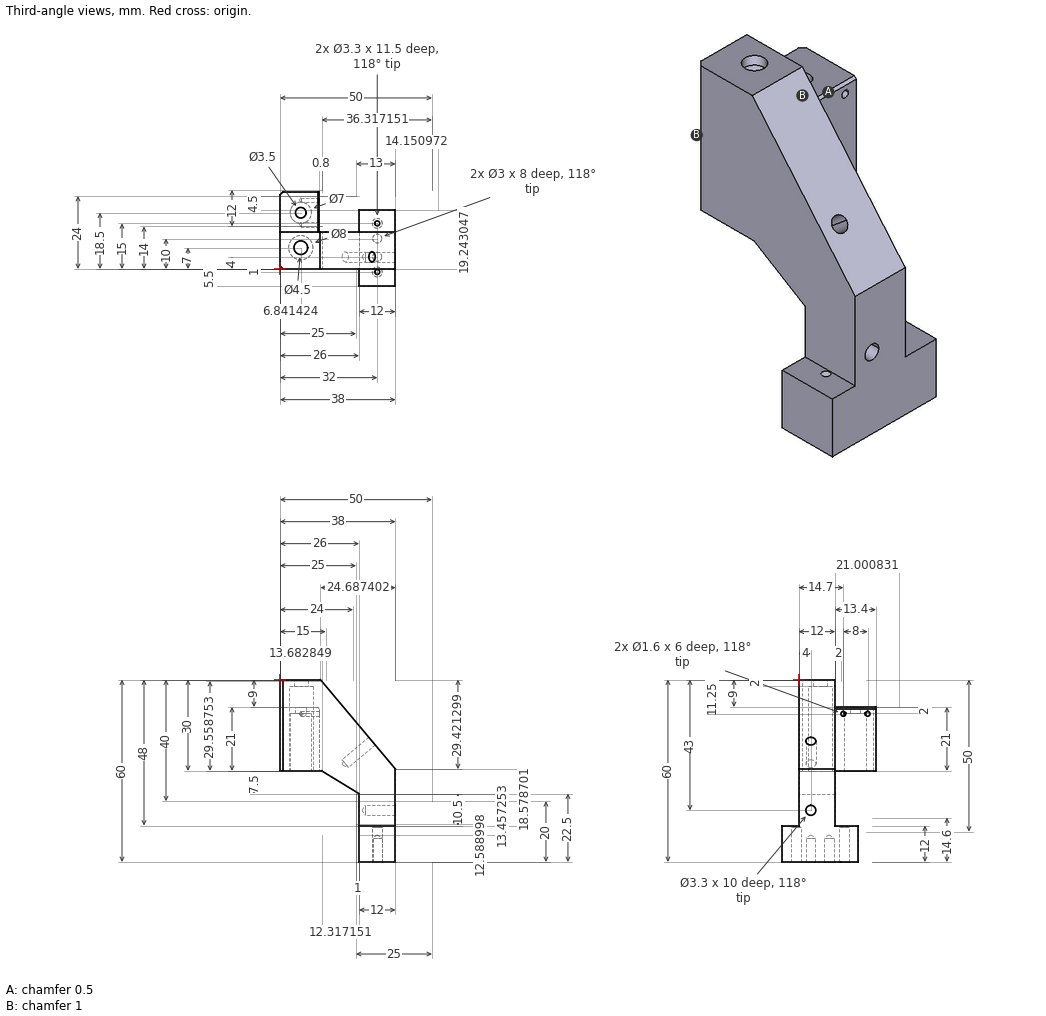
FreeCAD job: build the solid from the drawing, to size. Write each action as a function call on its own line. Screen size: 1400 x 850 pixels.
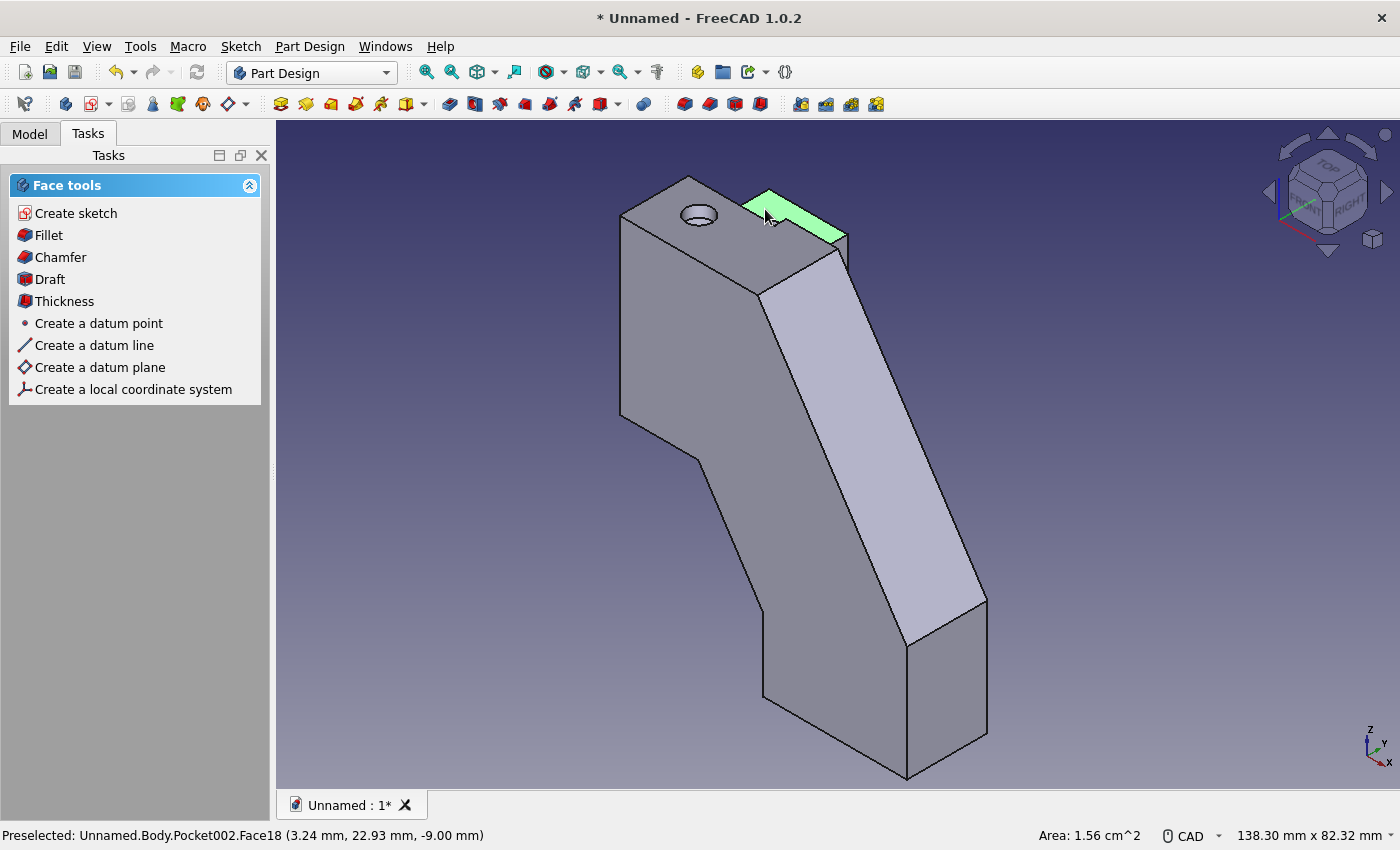
click(90, 104)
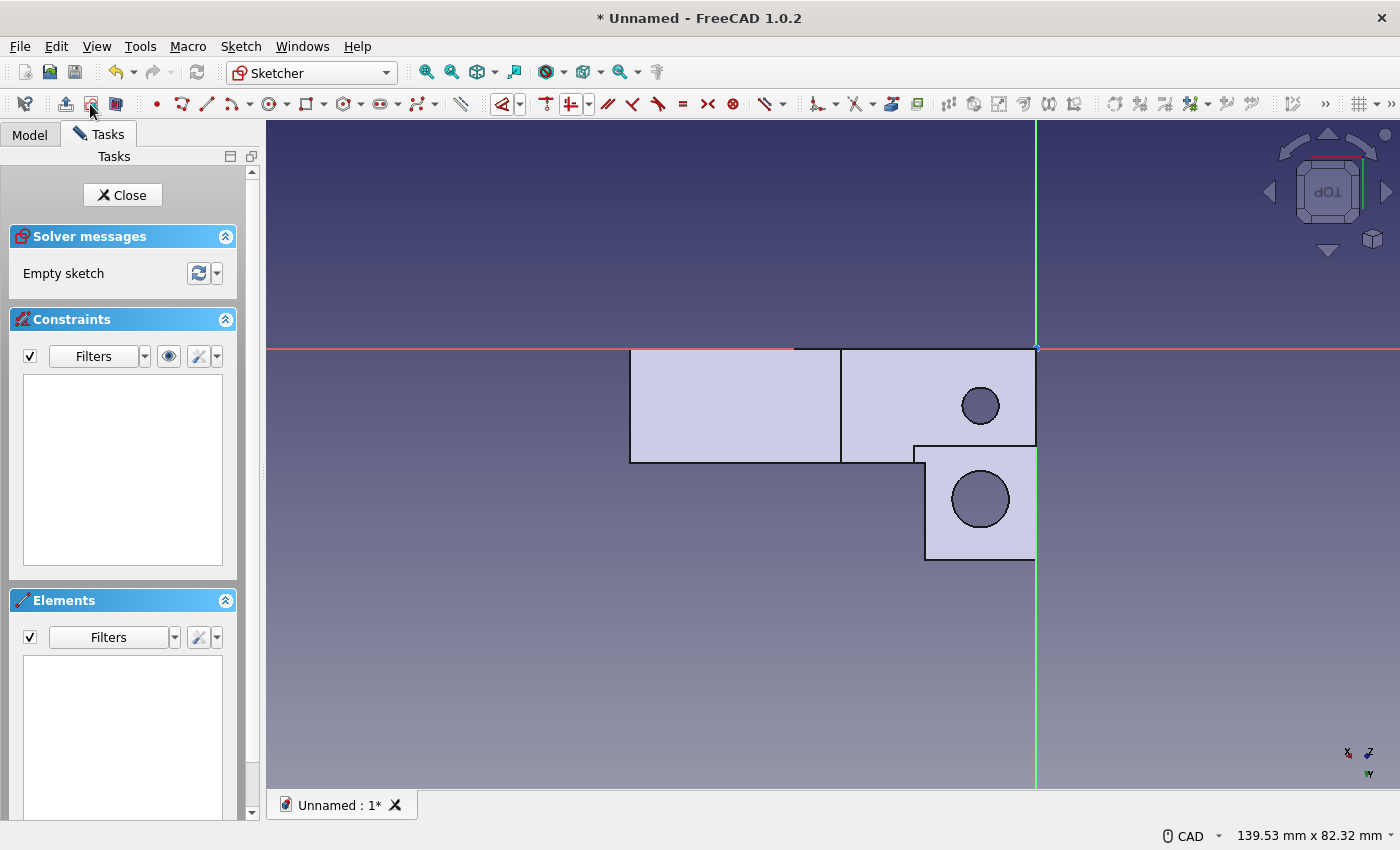
key(q)
key(s)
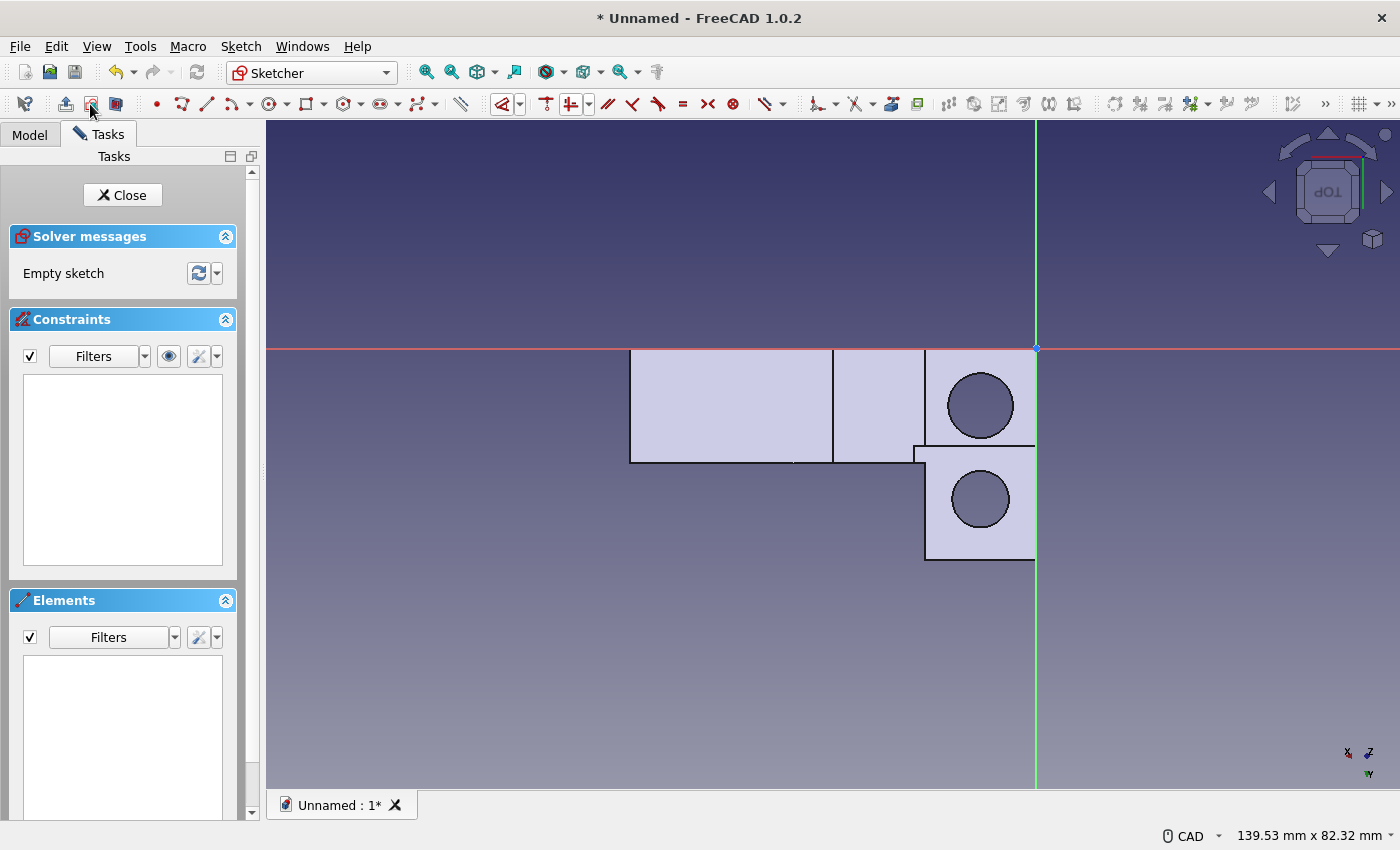
scroll(1014, 506, up, 10)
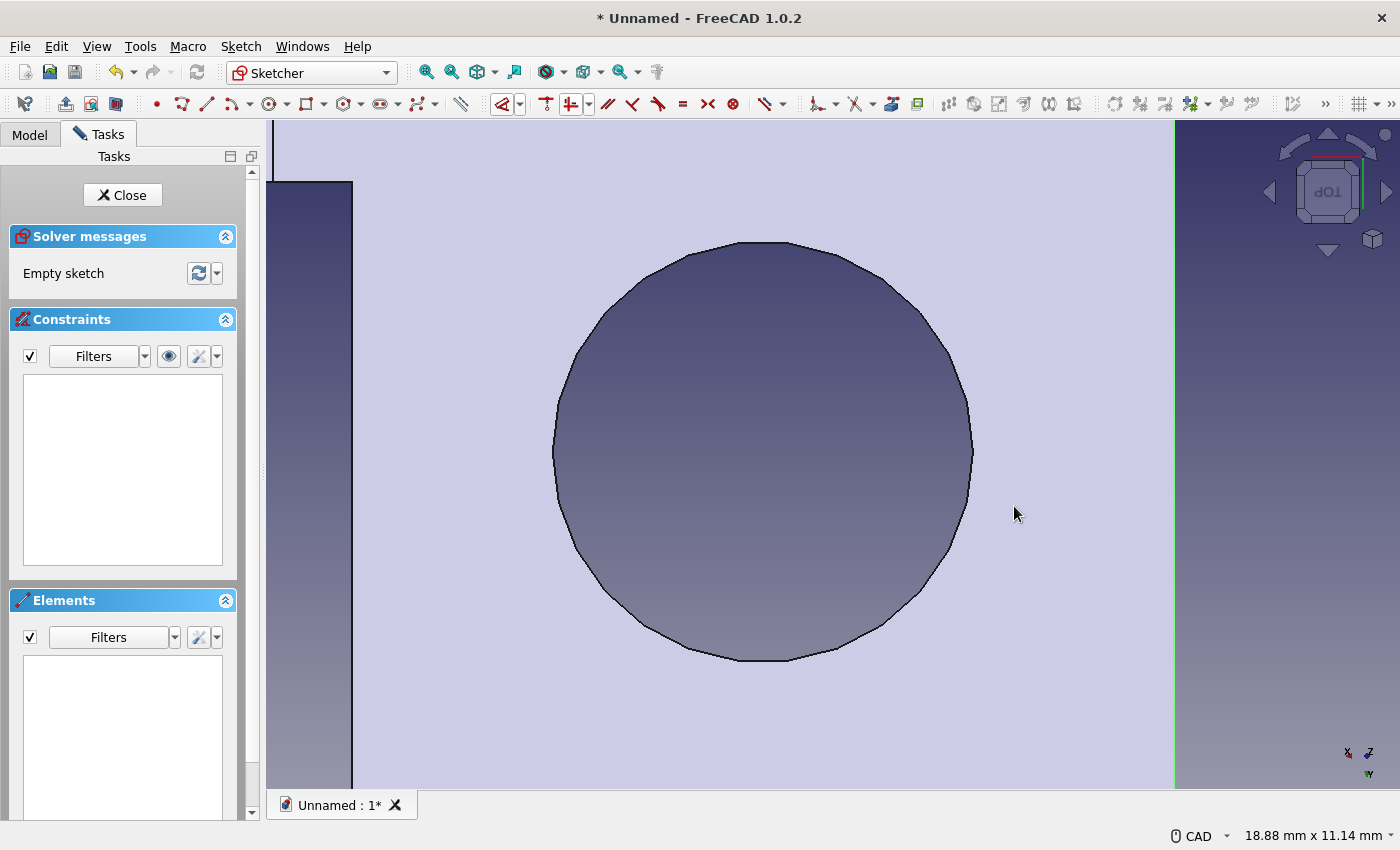
click(268, 104)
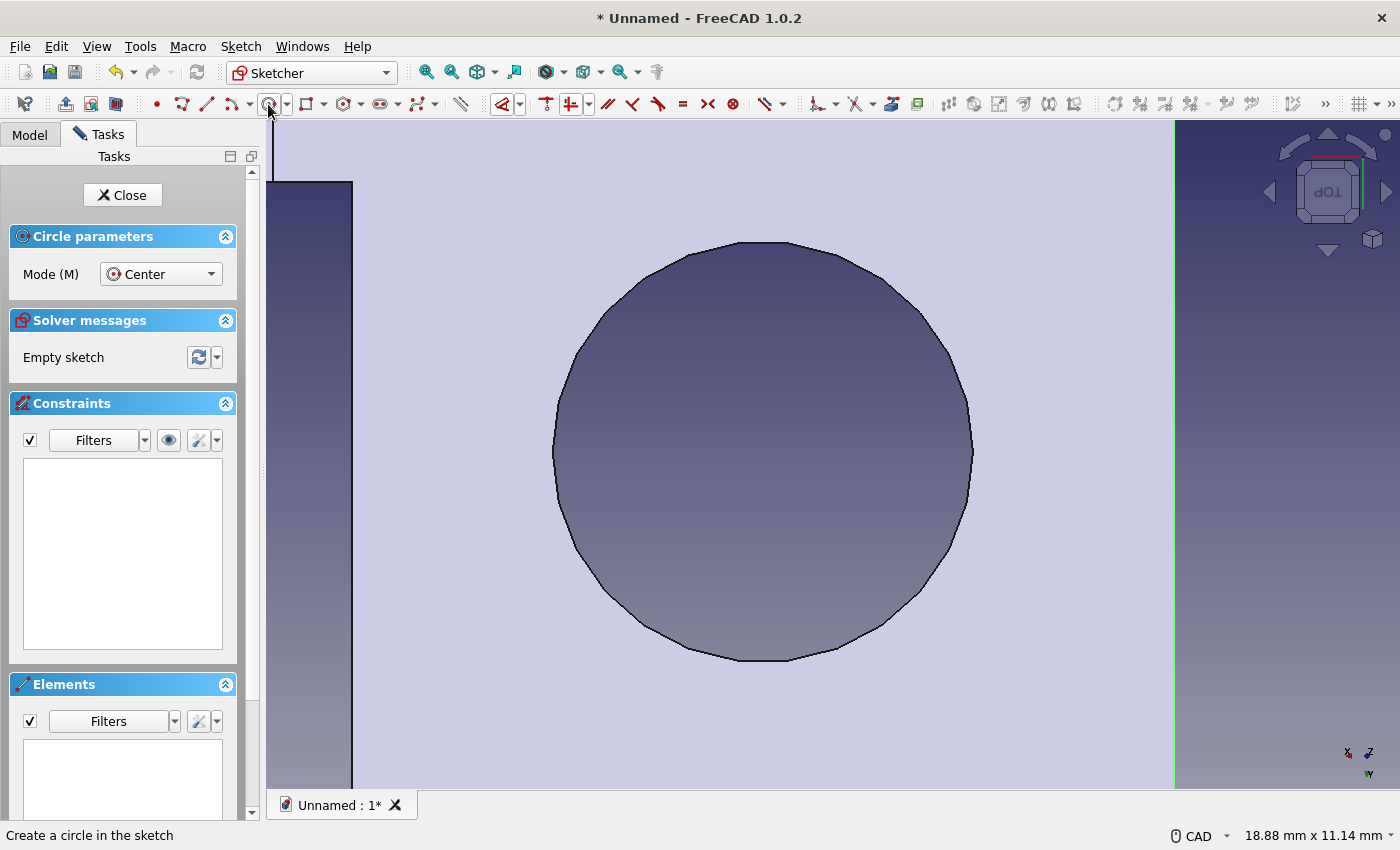
click(763, 452)
click(911, 303)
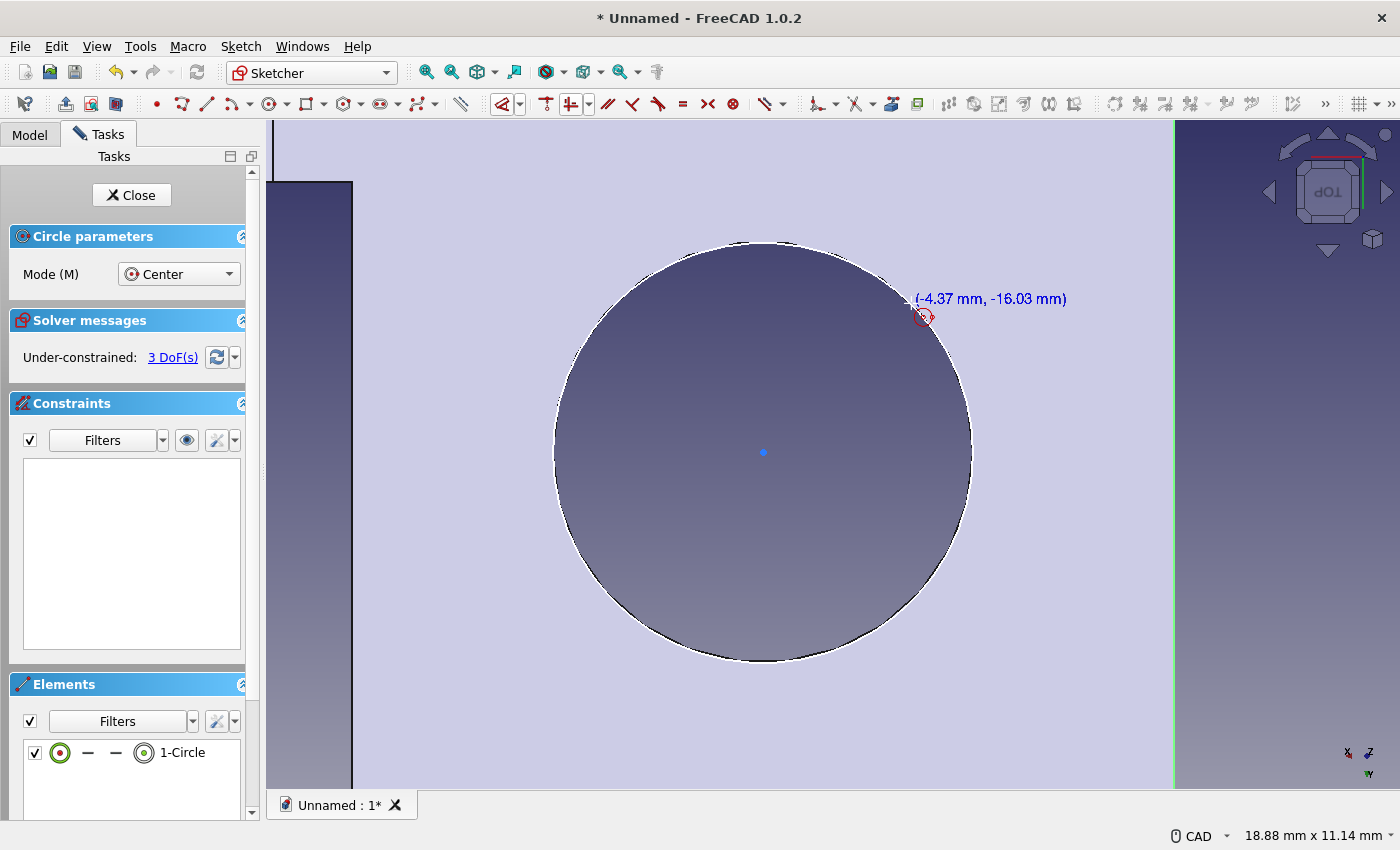
click(763, 453)
click(837, 378)
key(Escape)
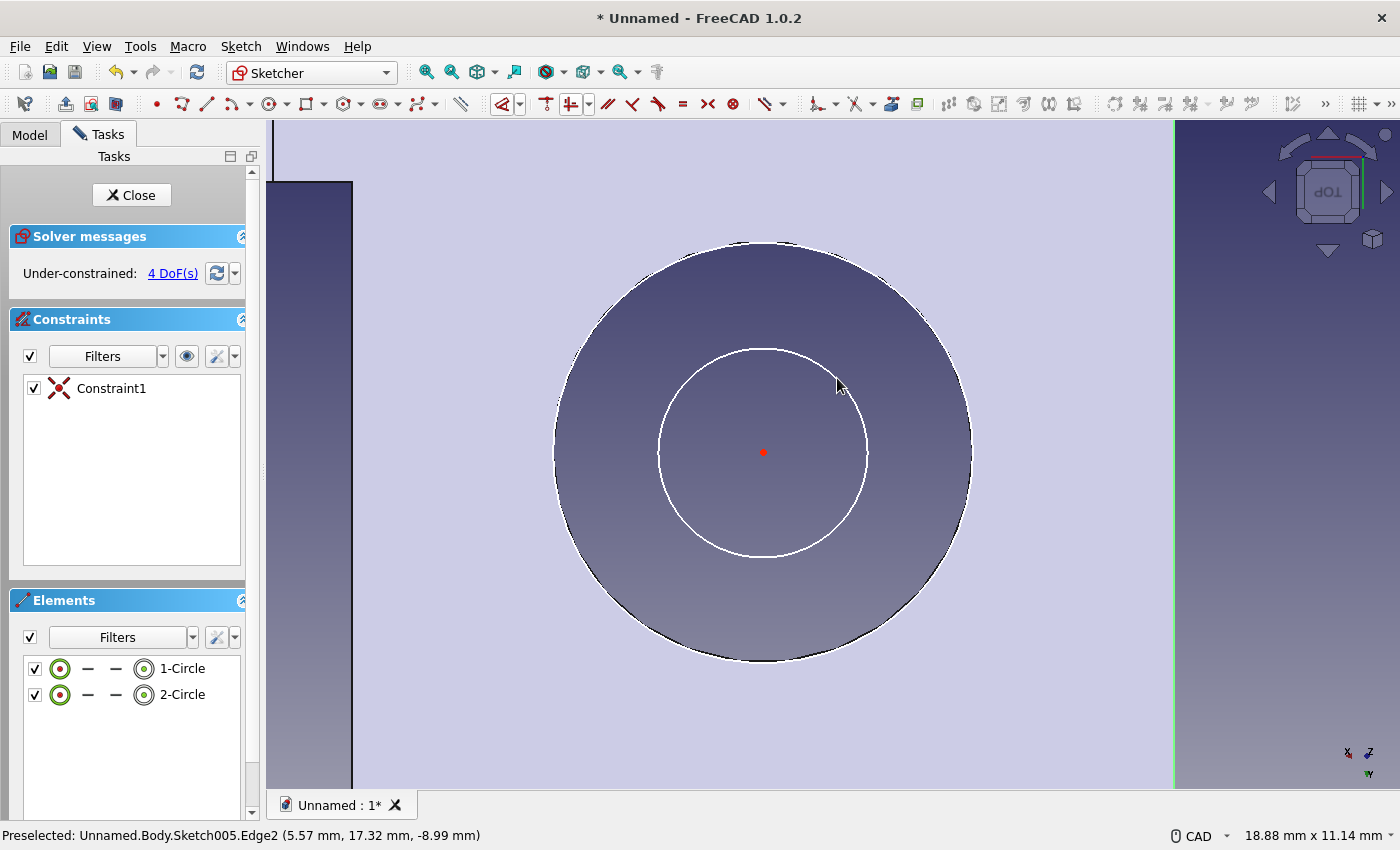
click(911, 304)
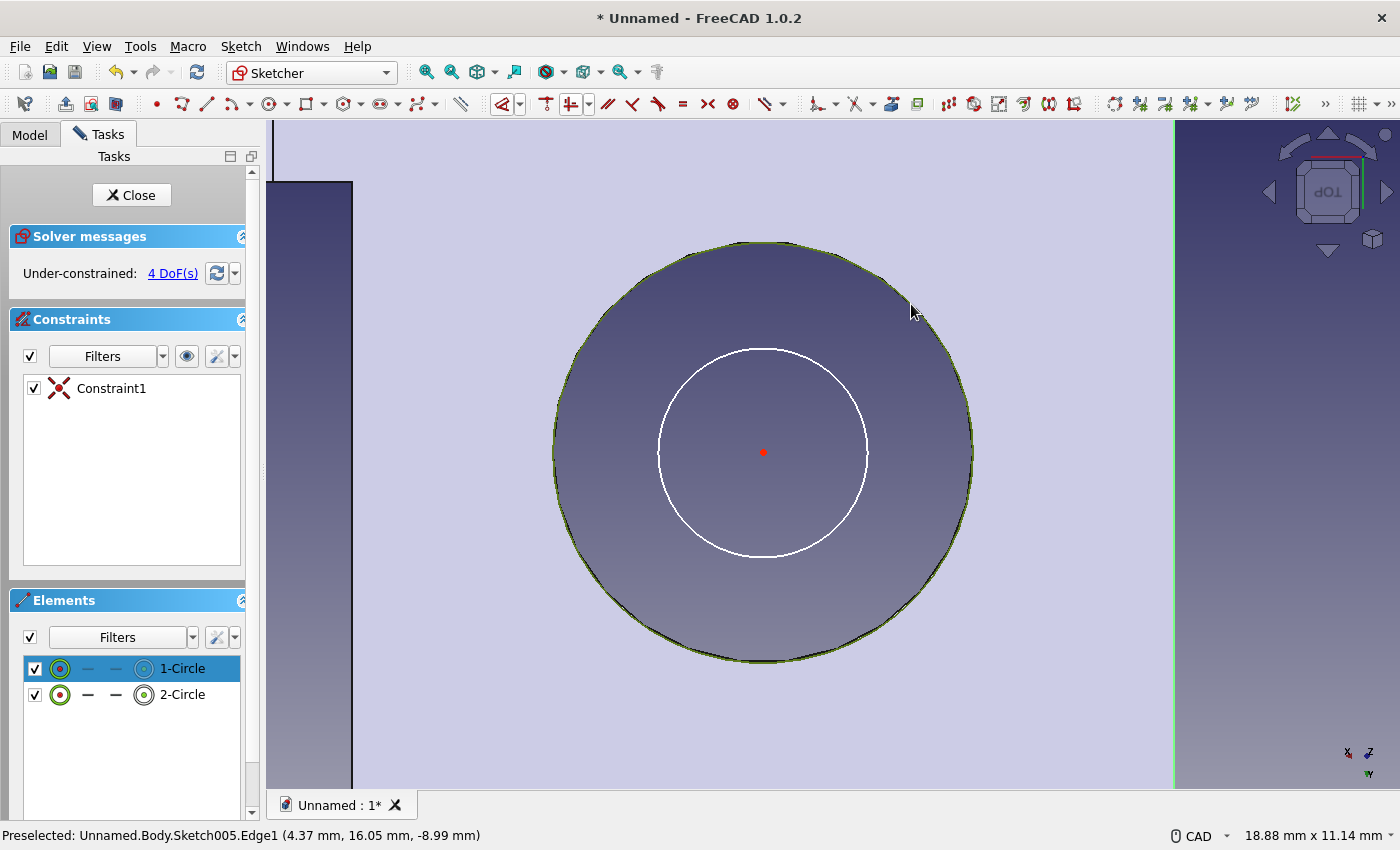
click(520, 104)